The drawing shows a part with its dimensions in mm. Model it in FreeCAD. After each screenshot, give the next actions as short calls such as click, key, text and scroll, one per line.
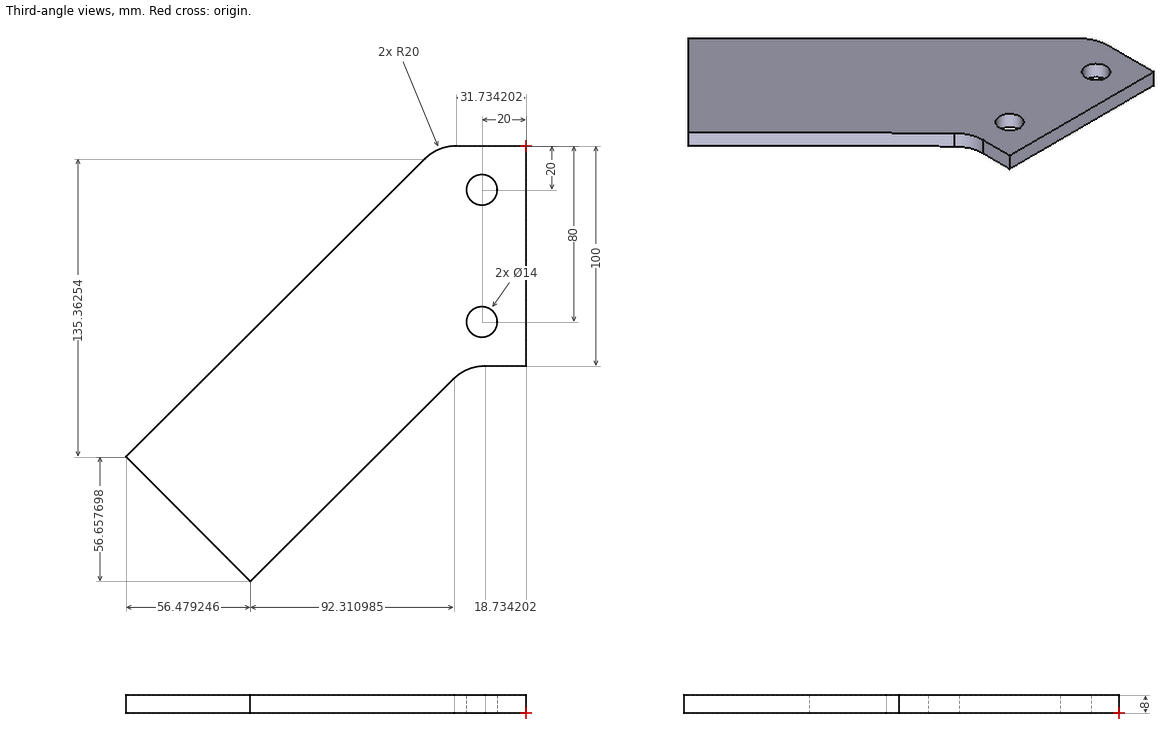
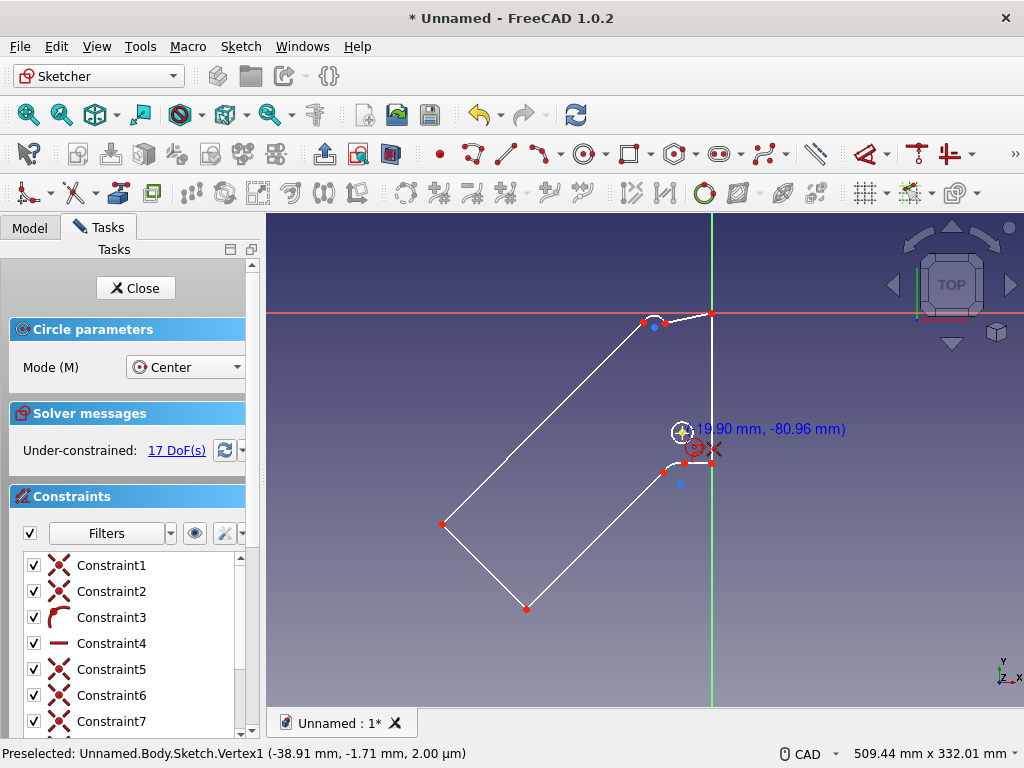
scroll(682, 343, up, 4)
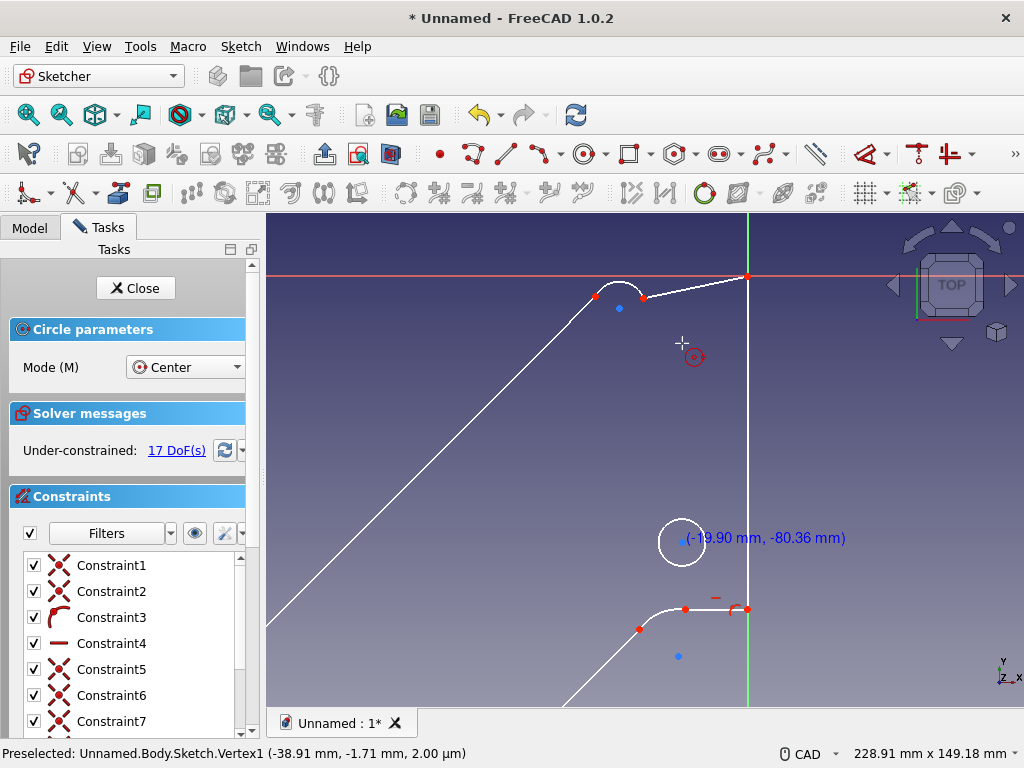
click(682, 343)
click(698, 326)
key(Escape)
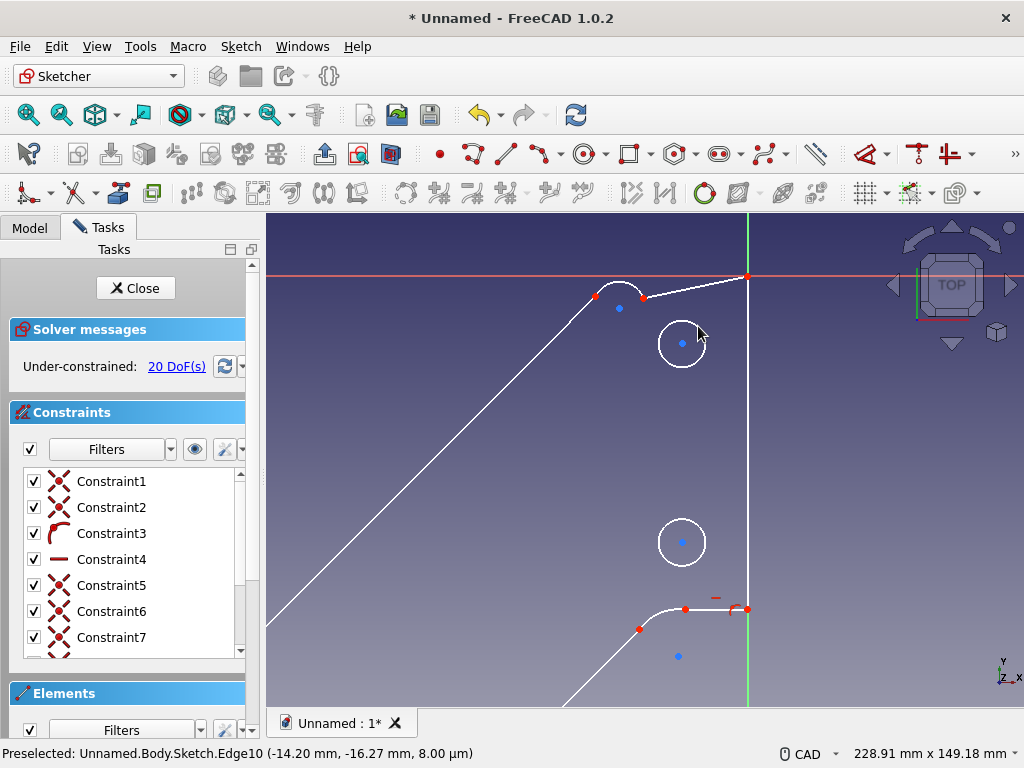
click(461, 431)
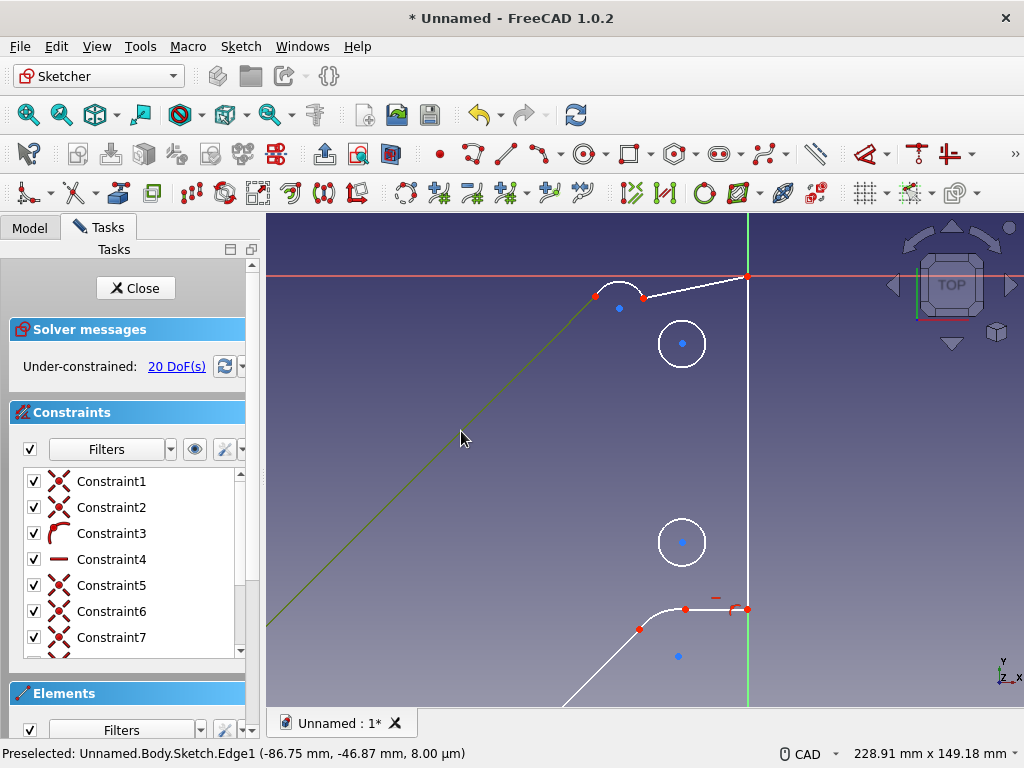
click(637, 288)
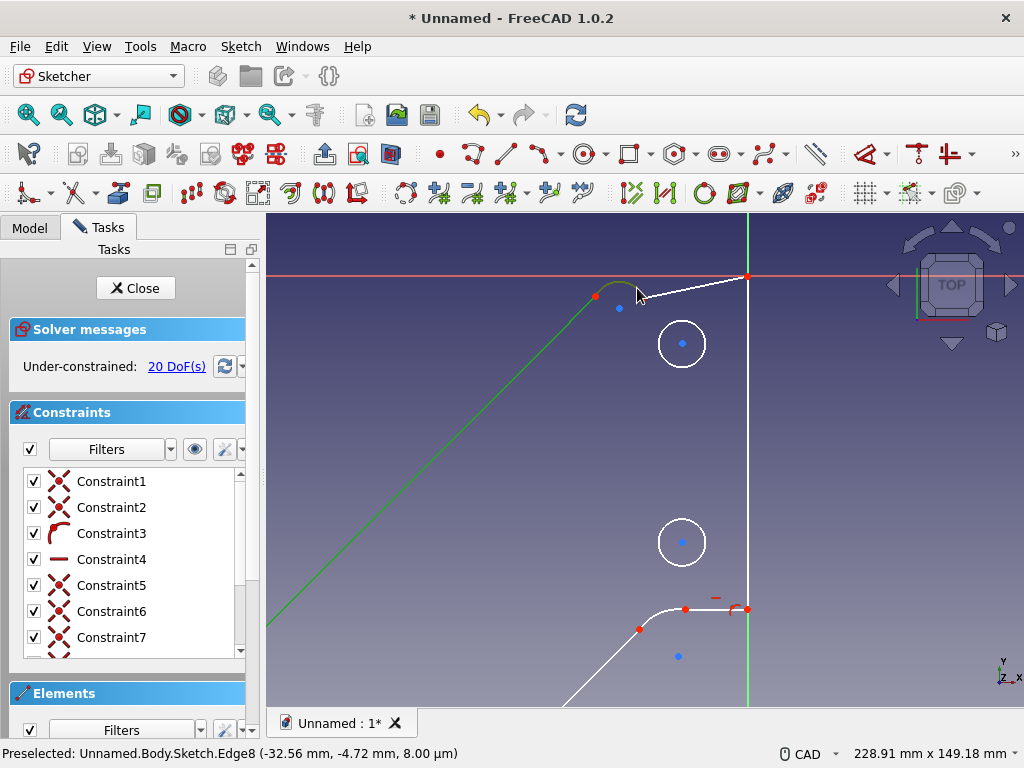
key(t)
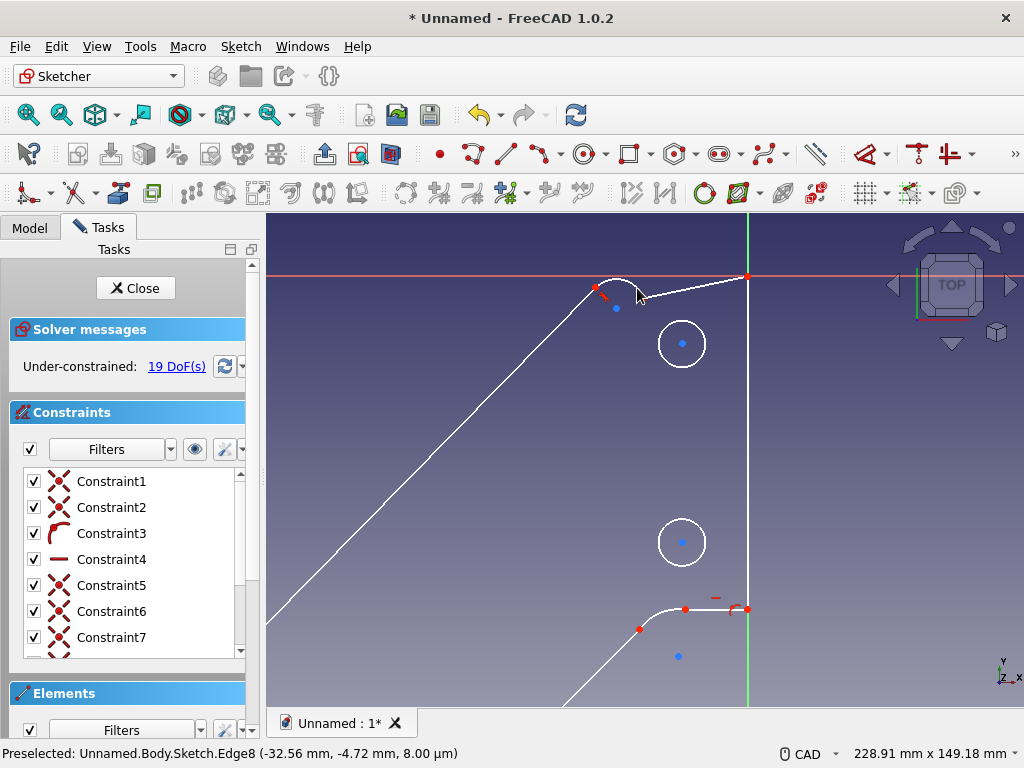
scroll(682, 342, down, 4)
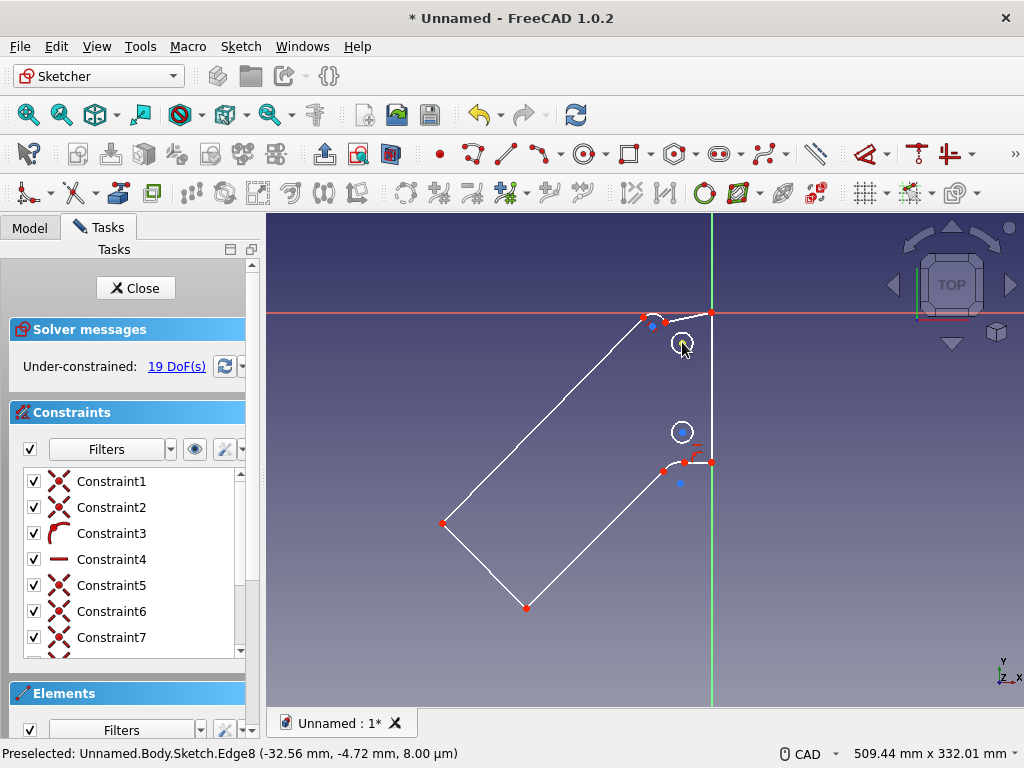
click(567, 567)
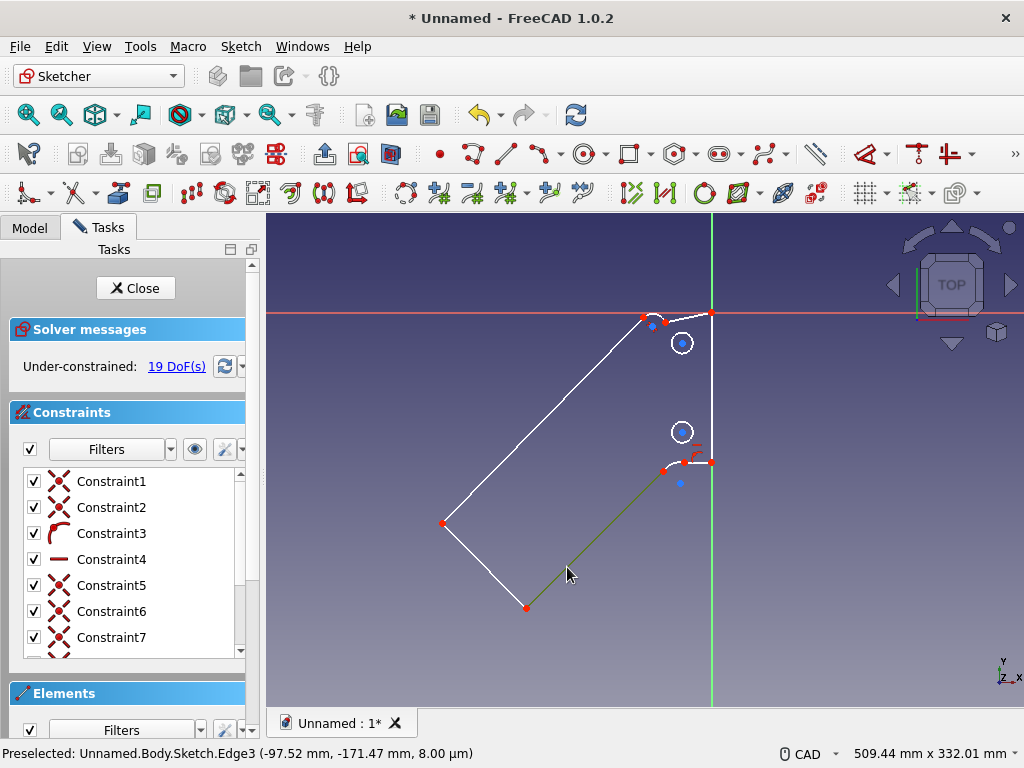
click(672, 464)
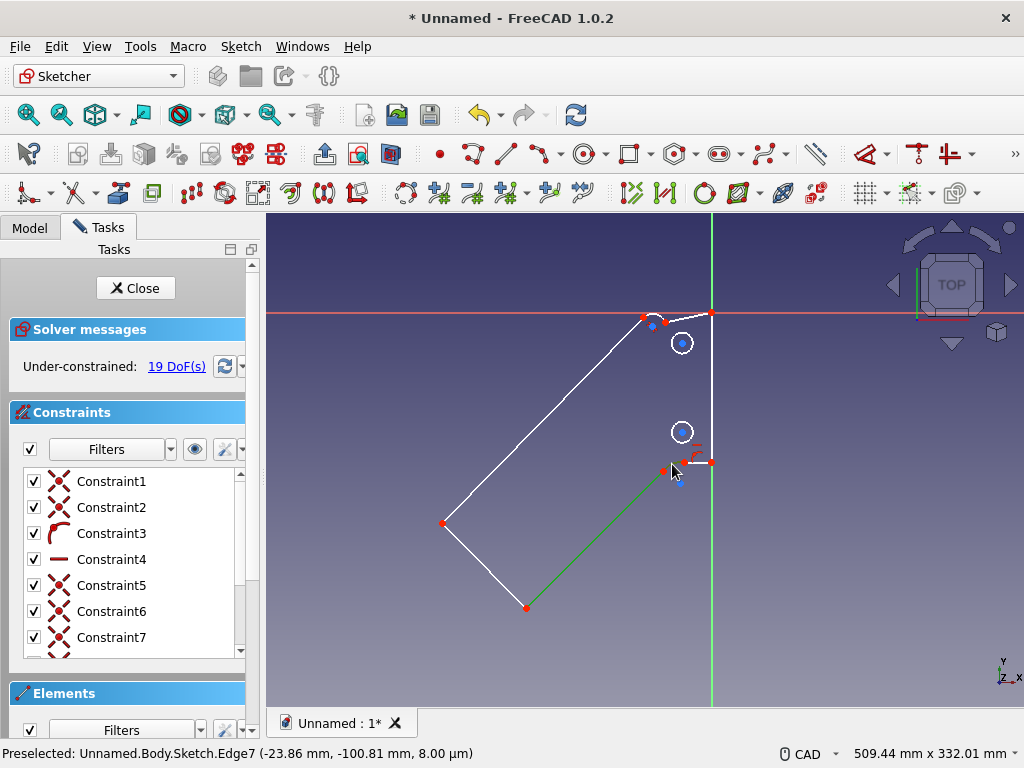
key(t)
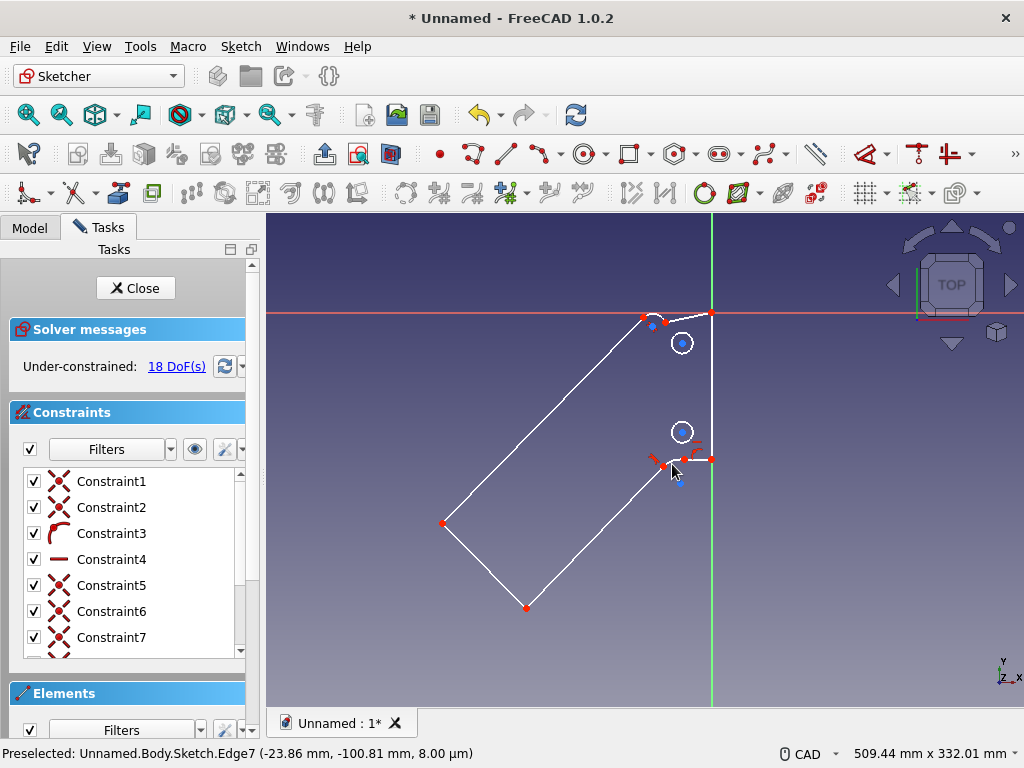
scroll(695, 460, up, 2)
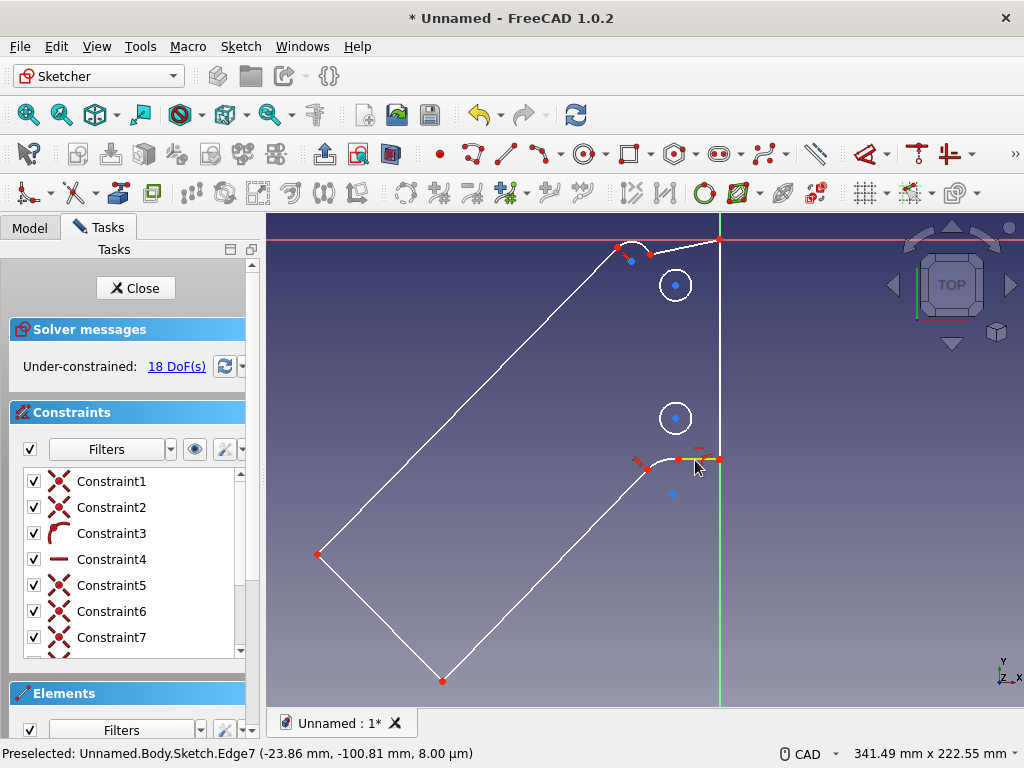
click(695, 459)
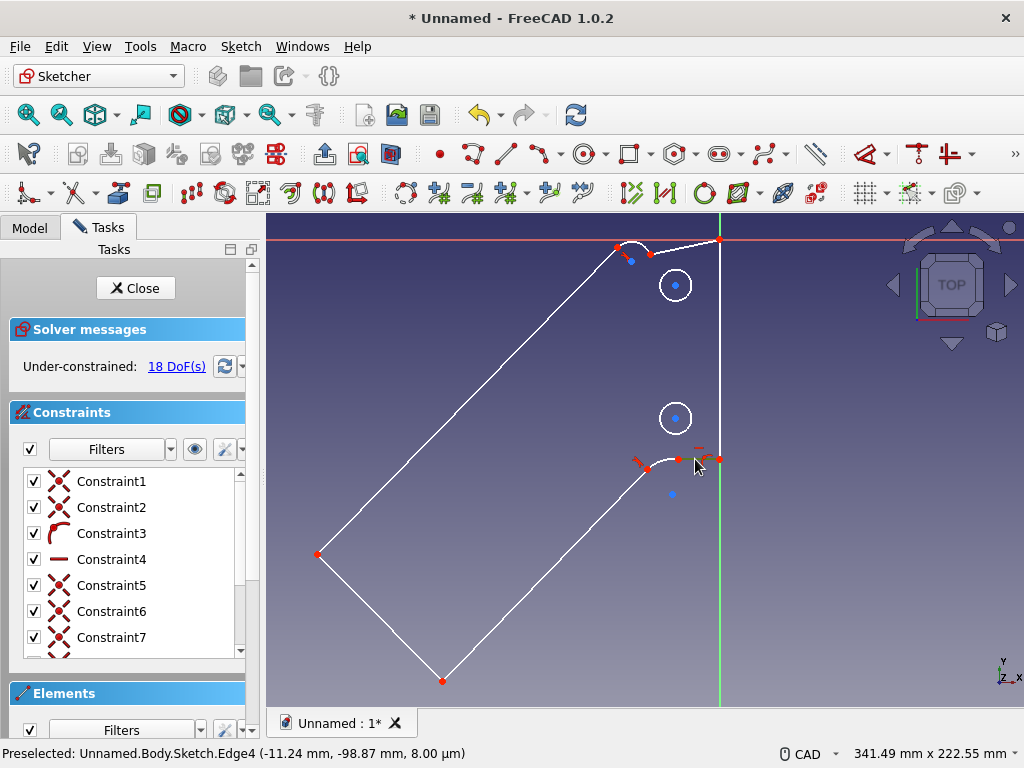
scroll(668, 459, up, 2)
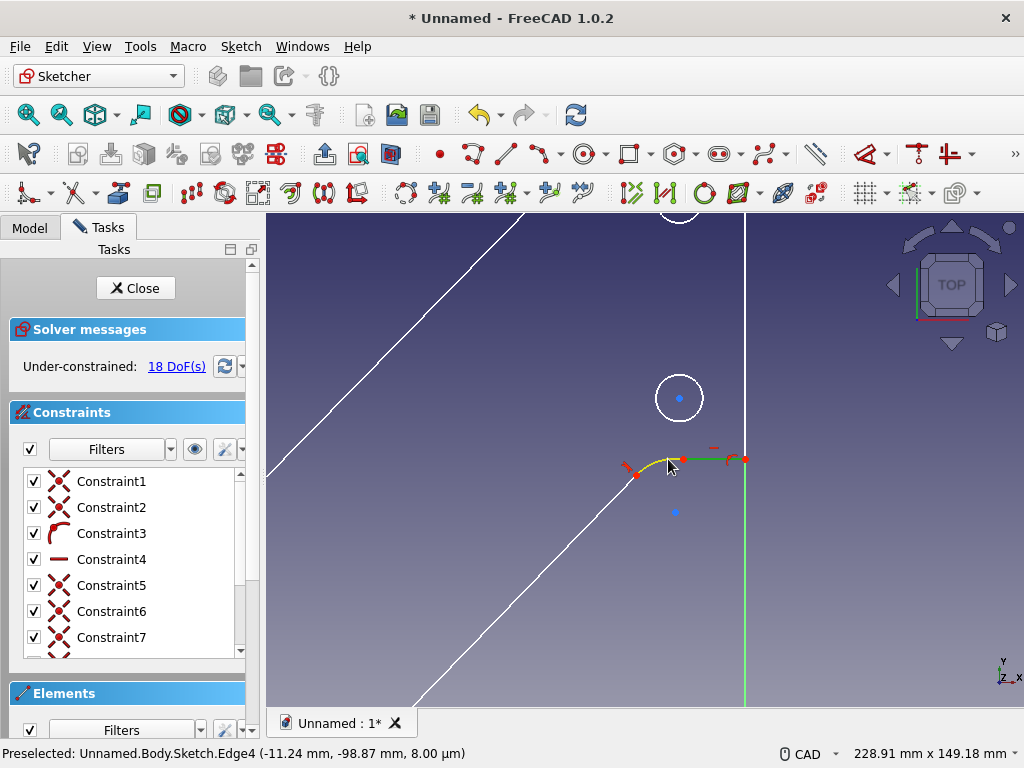
click(668, 459)